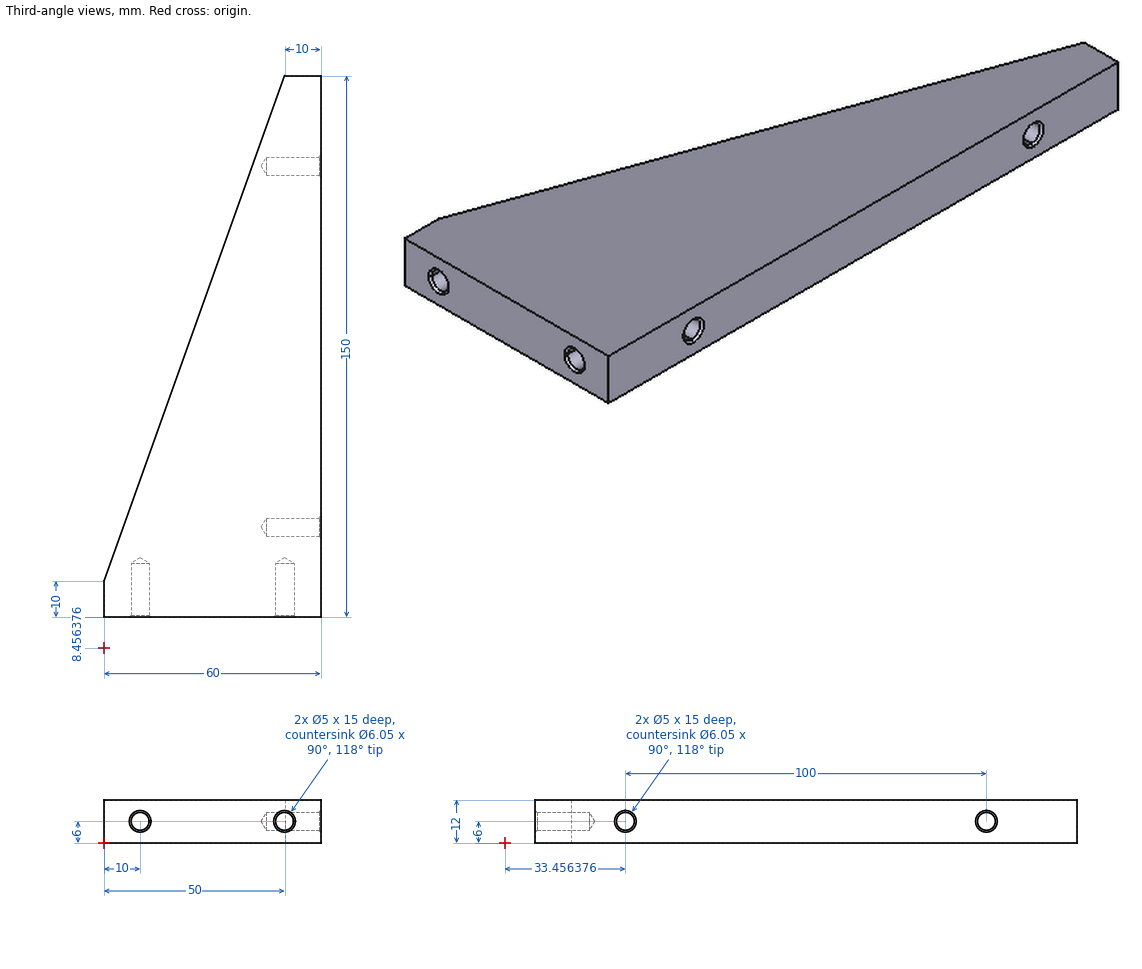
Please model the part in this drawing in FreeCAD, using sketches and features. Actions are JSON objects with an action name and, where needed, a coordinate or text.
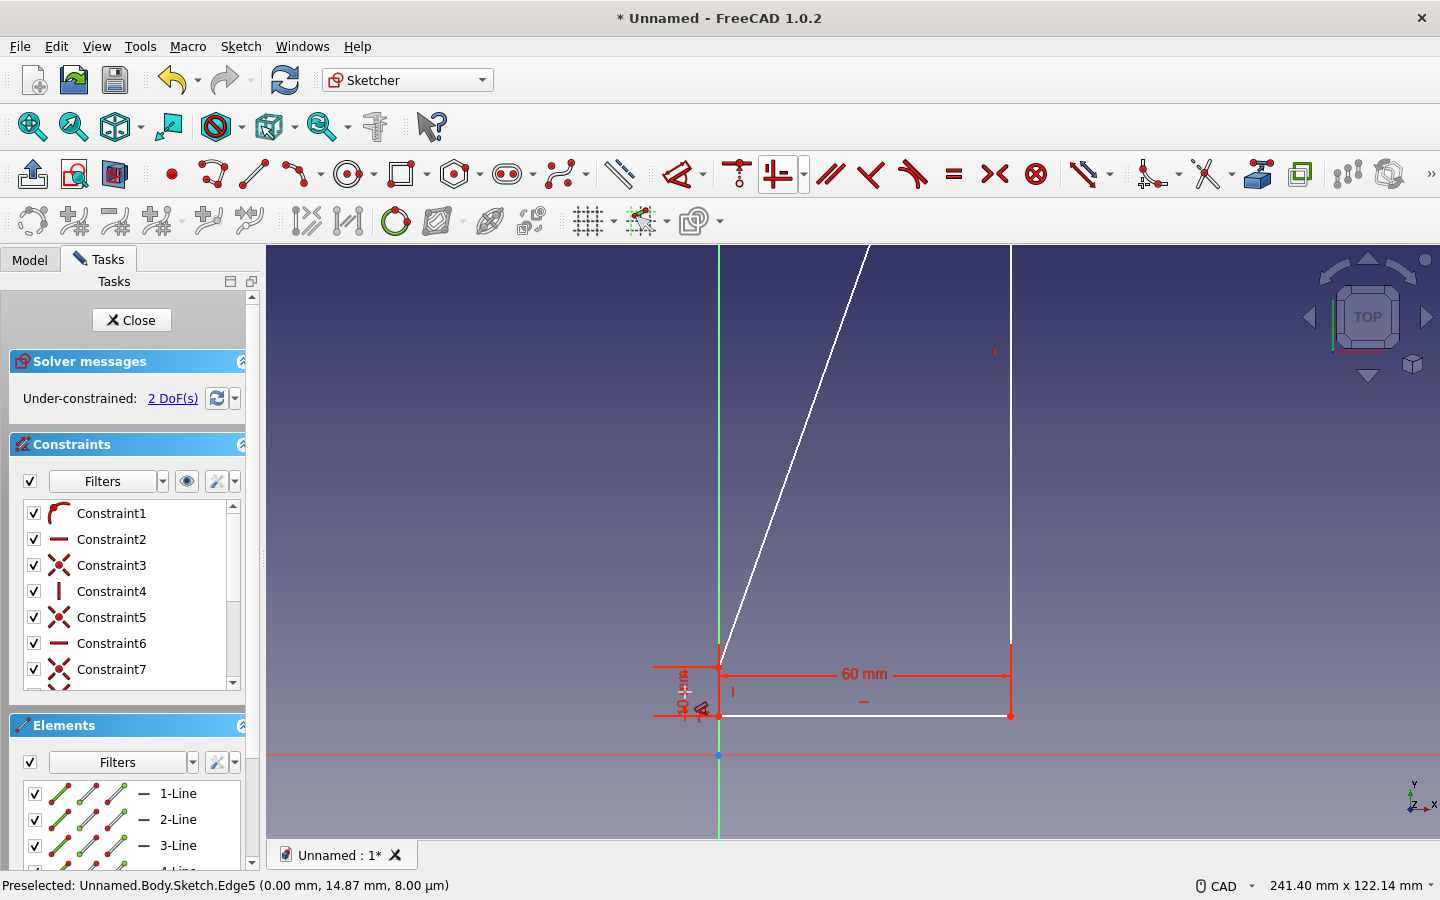
{"action": "left_click", "coordinate": [1011, 497]}
{"action": "left_click", "coordinate": [1045, 495]}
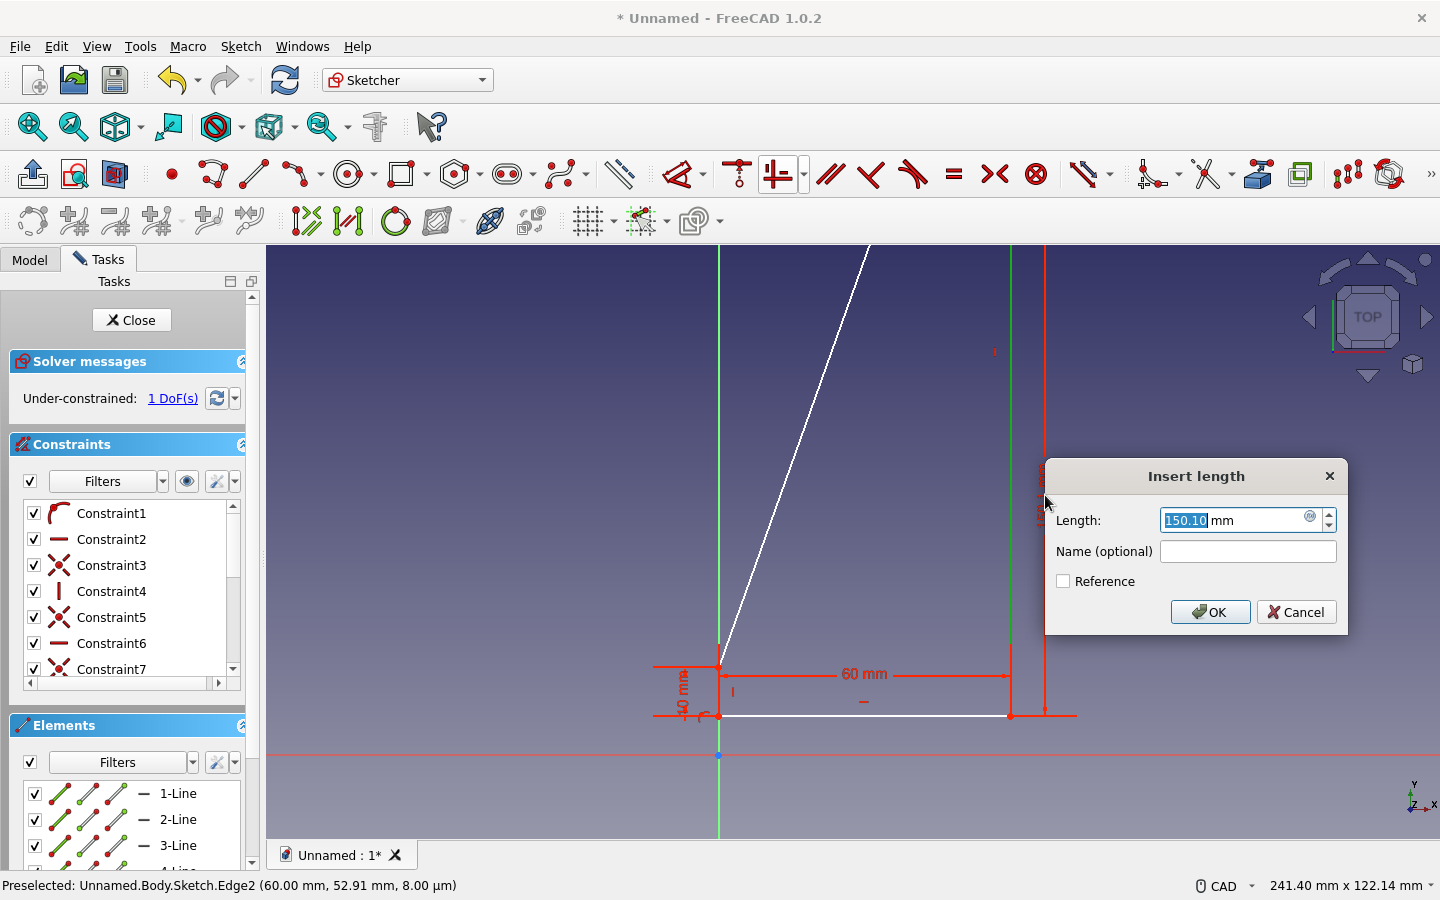
{"action": "type", "text": "150"}
{"action": "key", "text": "Return"}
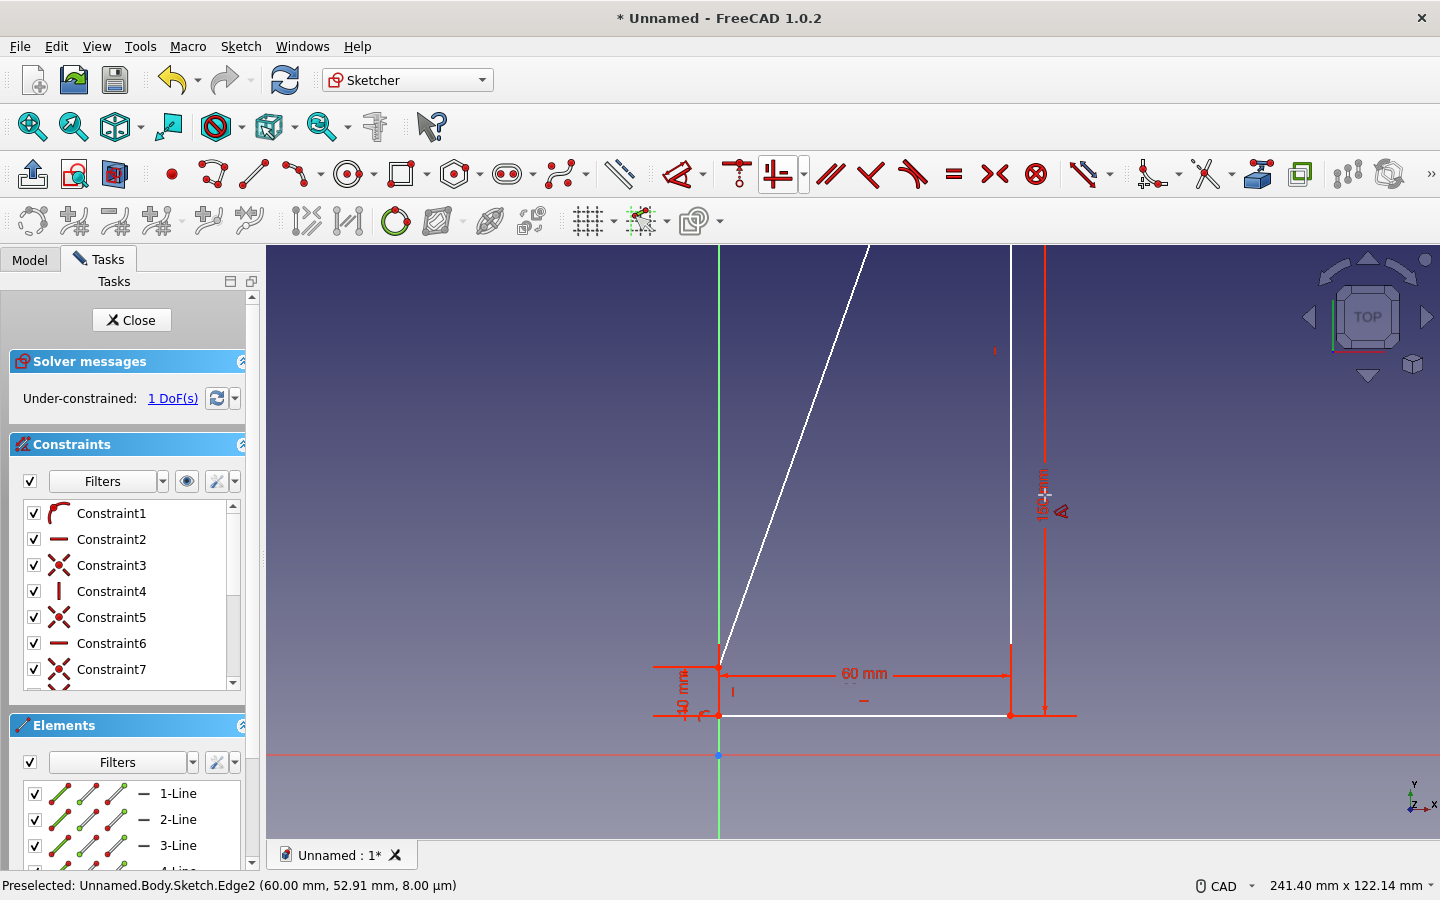
{"action": "left_click", "coordinate": [719, 716]}
{"action": "left_click", "coordinate": [685, 735]}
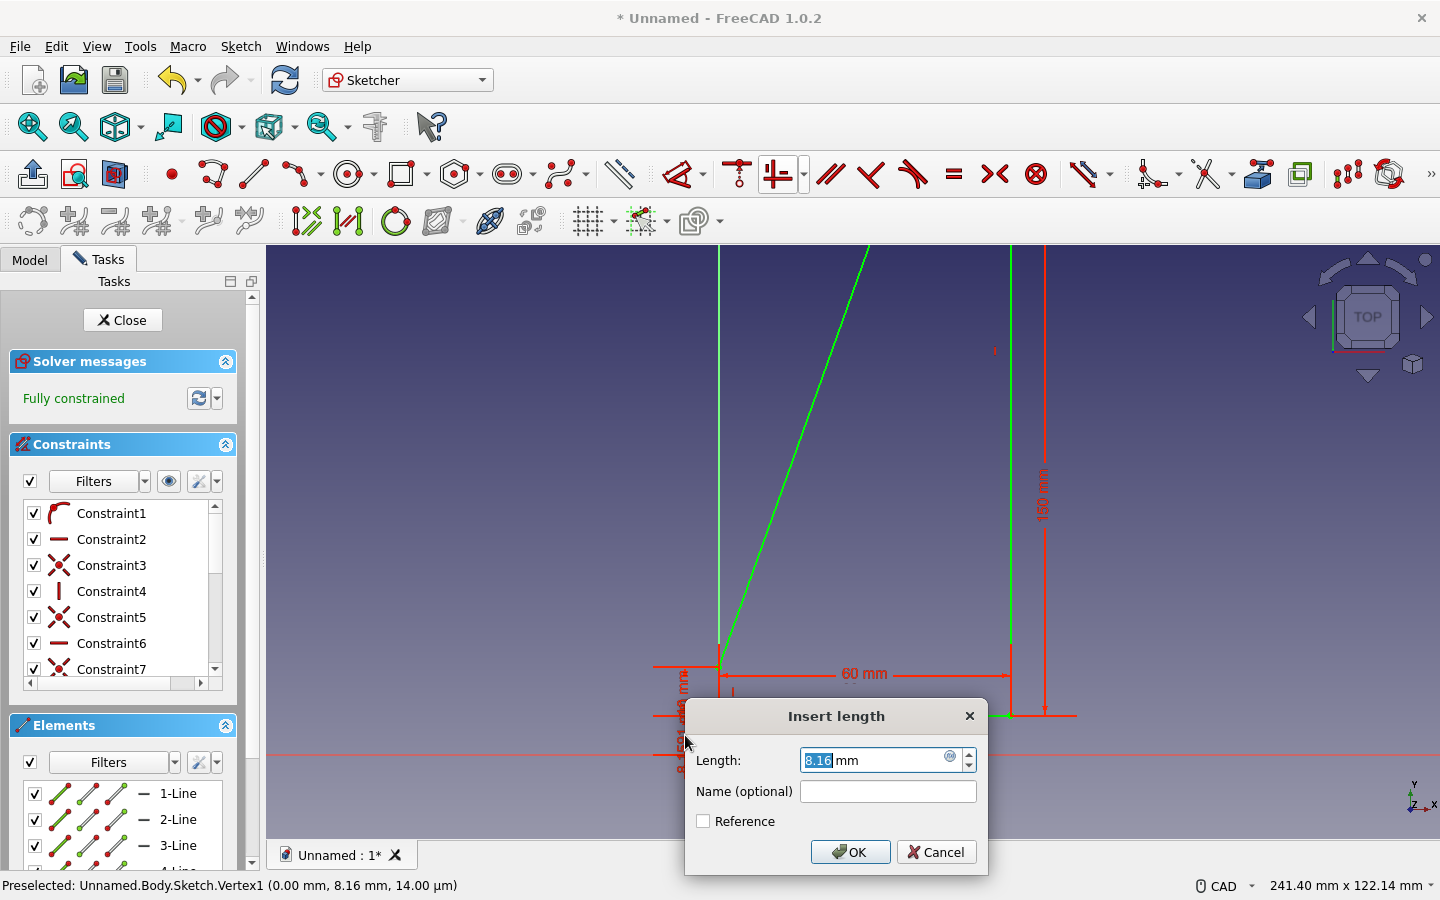
{"action": "type", "text": "8.456376"}
{"action": "key", "text": "Return"}
{"action": "key", "text": "Escape"}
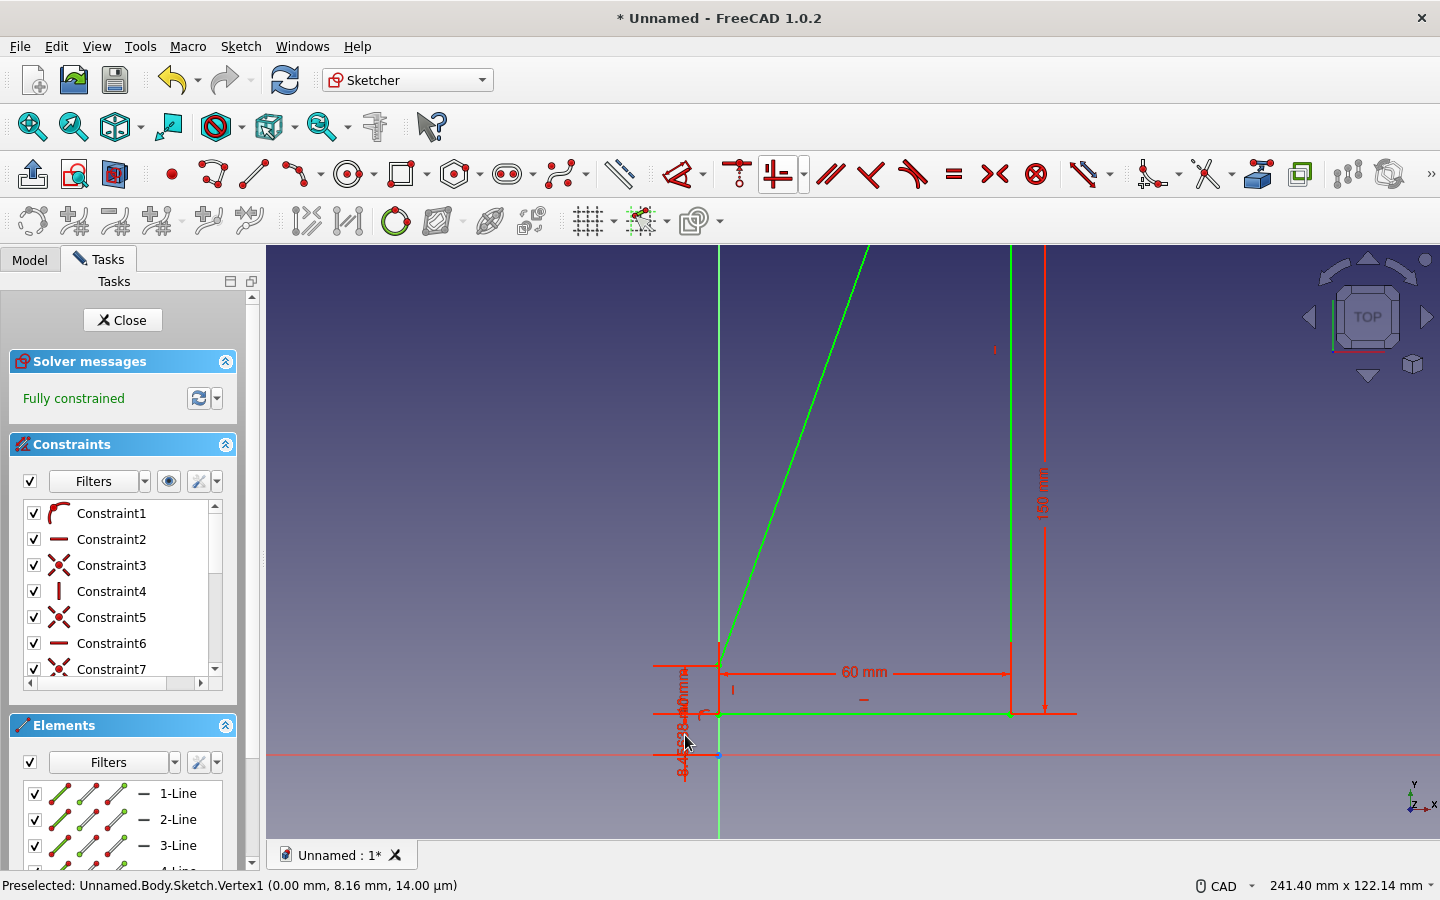
{"action": "left_click", "coordinate": [123, 320]}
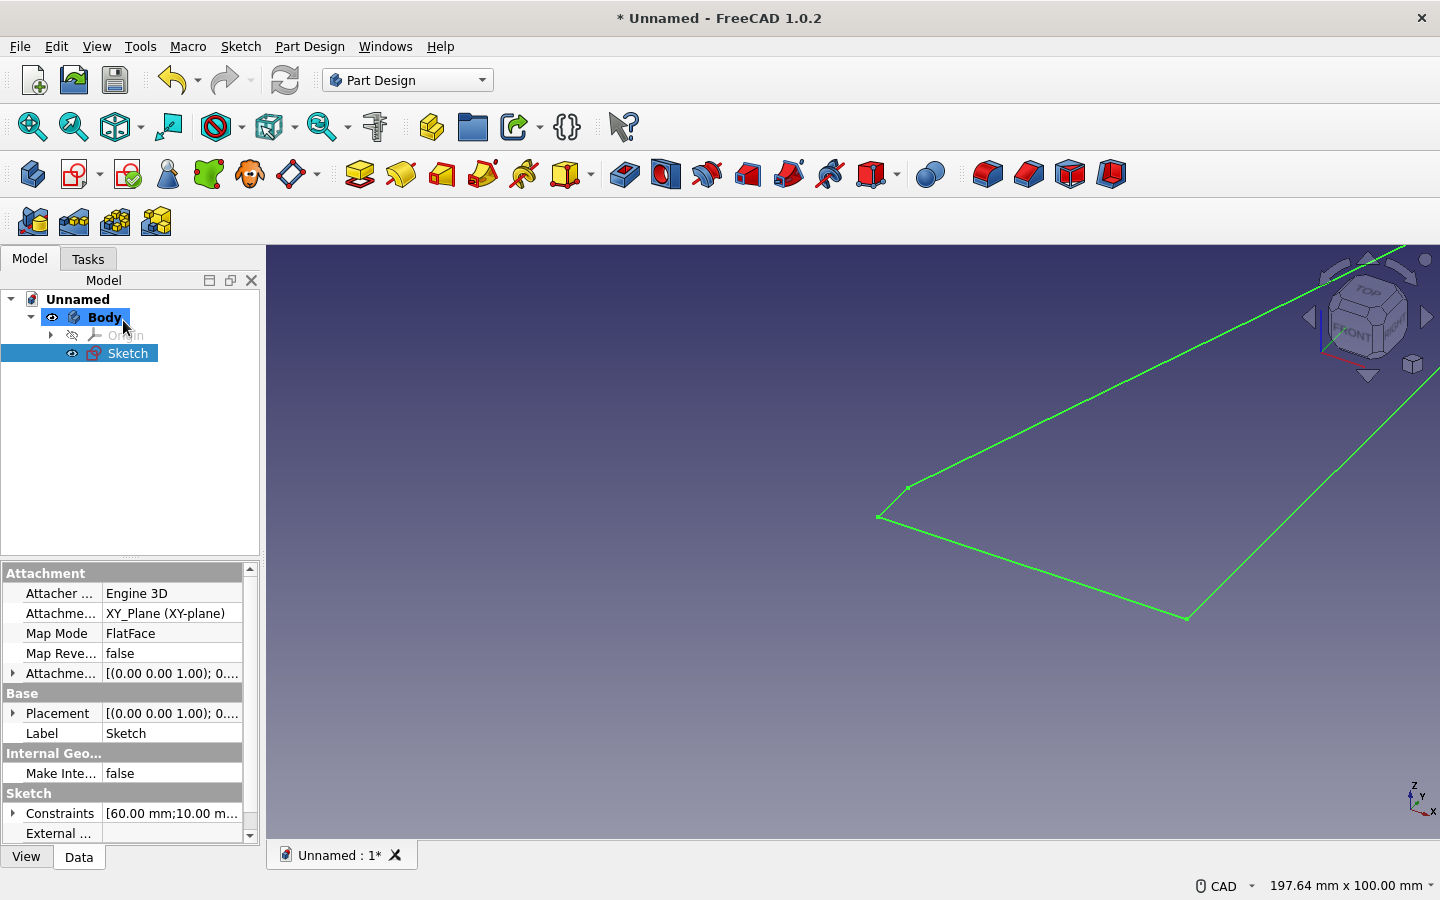
{"action": "left_click", "coordinate": [360, 174]}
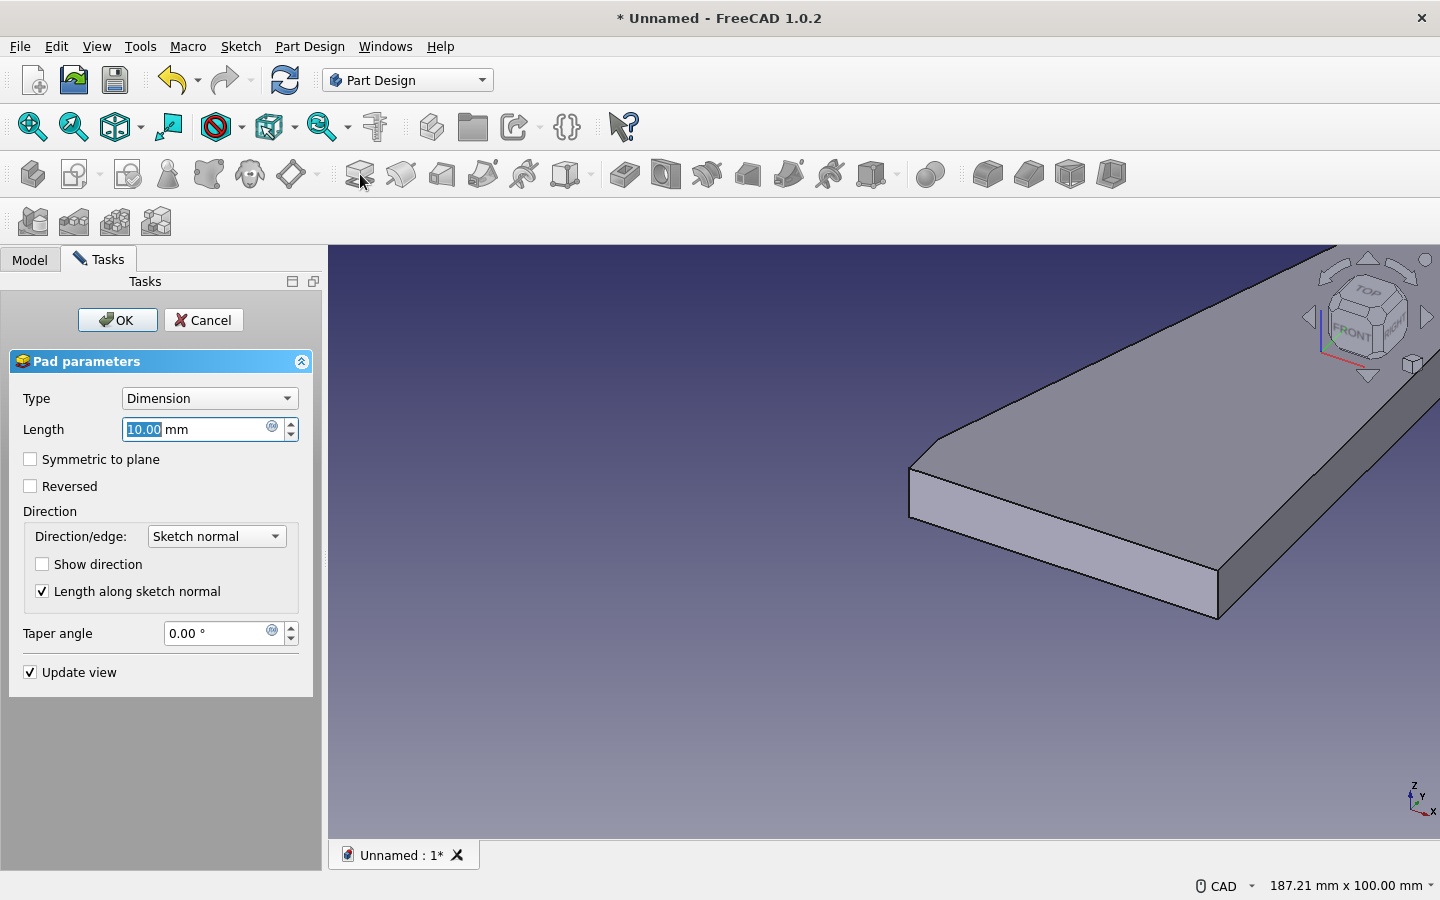
{"action": "type", "text": "12"}
{"action": "key", "text": "Tab"}